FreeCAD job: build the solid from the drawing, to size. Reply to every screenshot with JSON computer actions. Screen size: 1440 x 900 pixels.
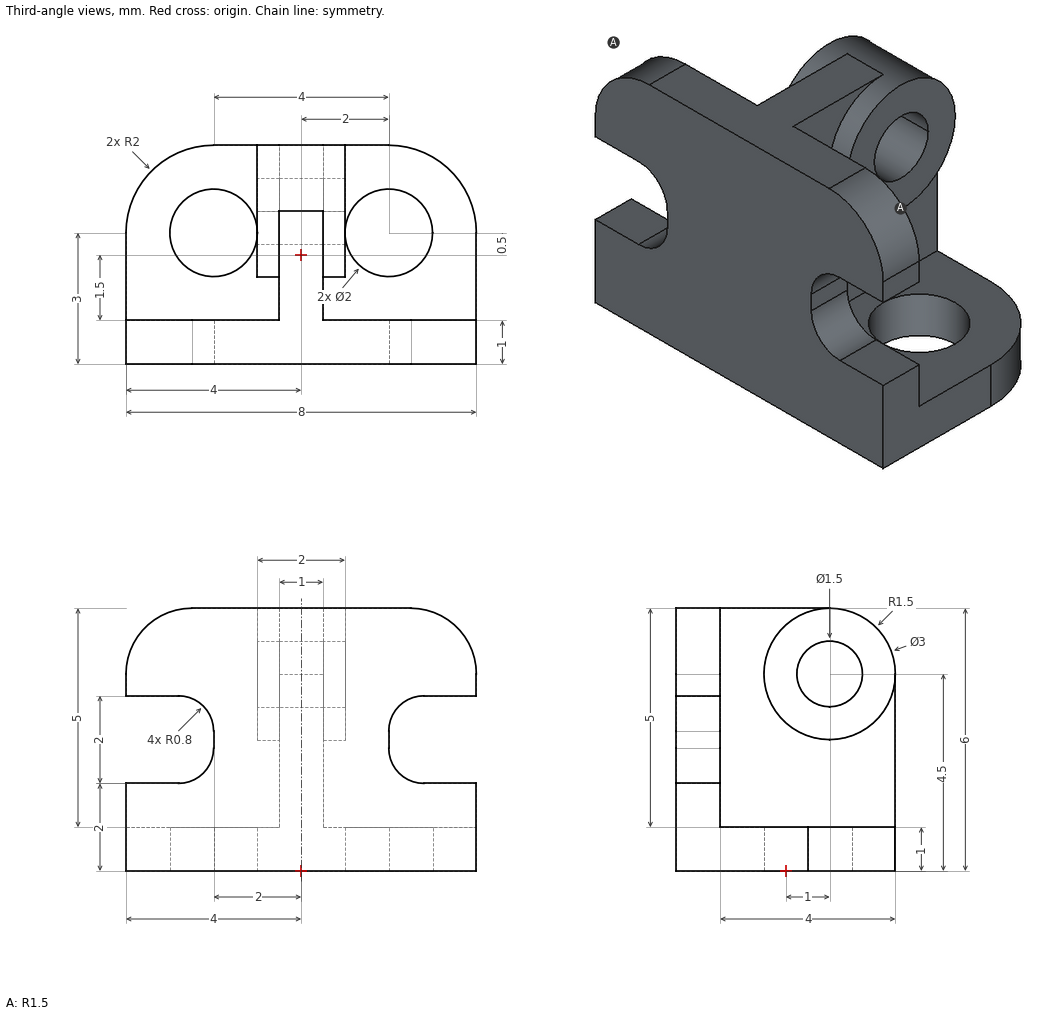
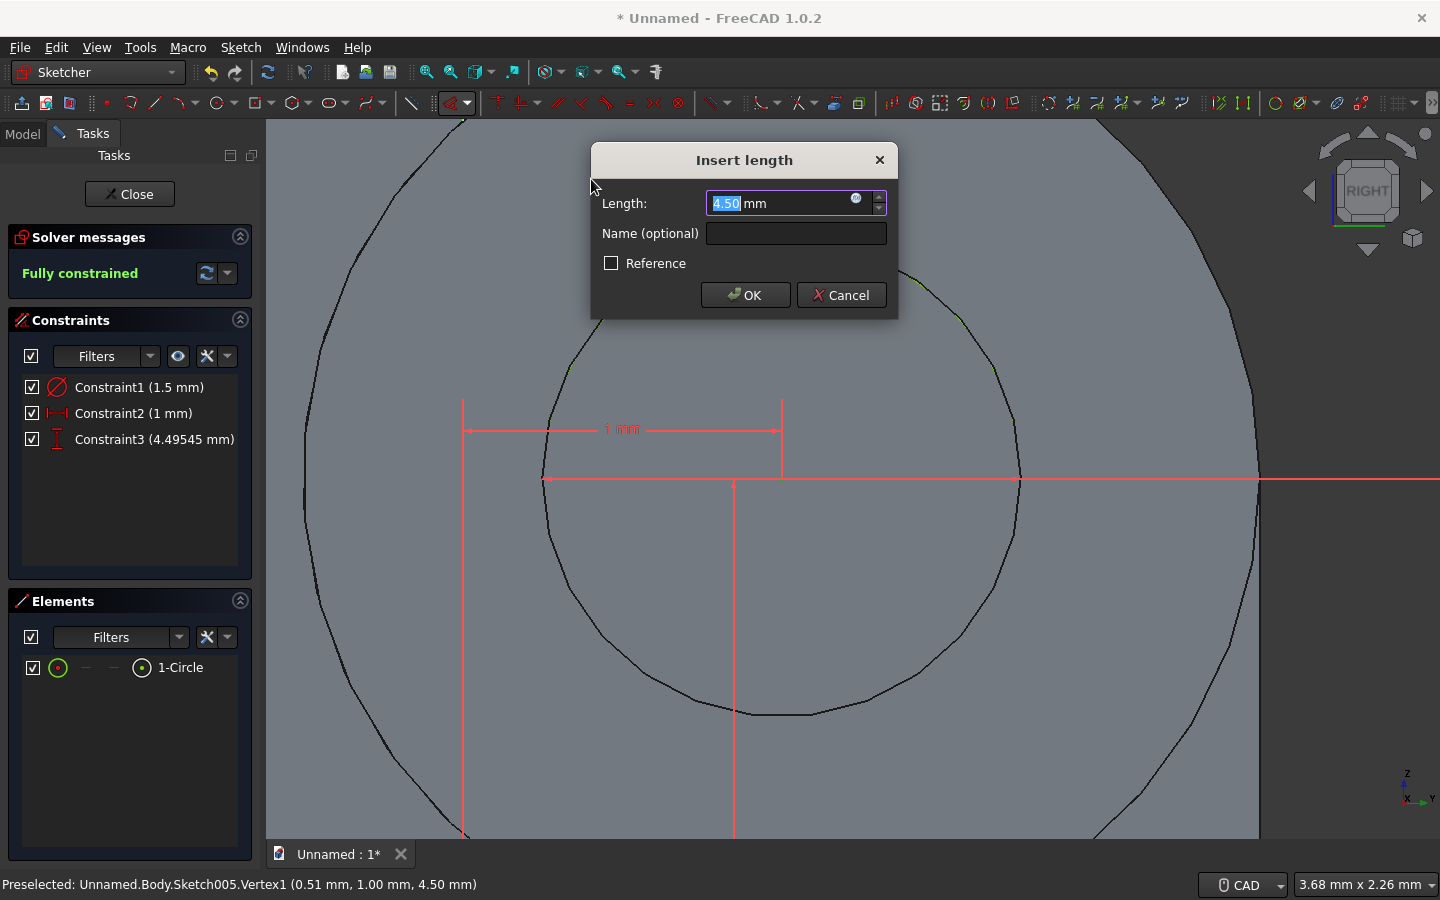
{"action": "type", "text": "4.5"}
{"action": "key", "text": "Return"}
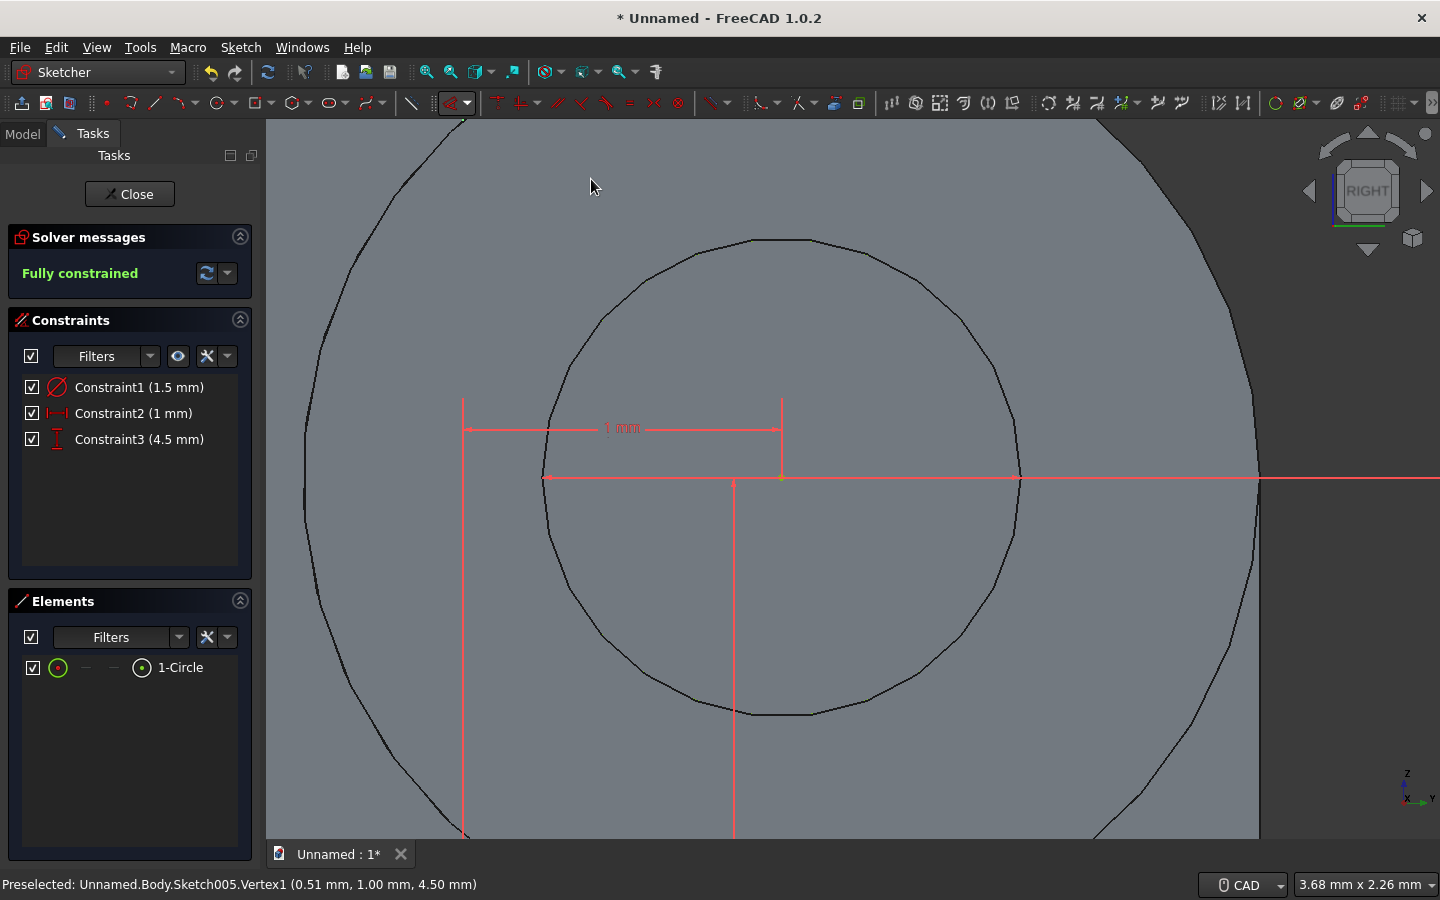
{"action": "left_click", "coordinate": [130, 194]}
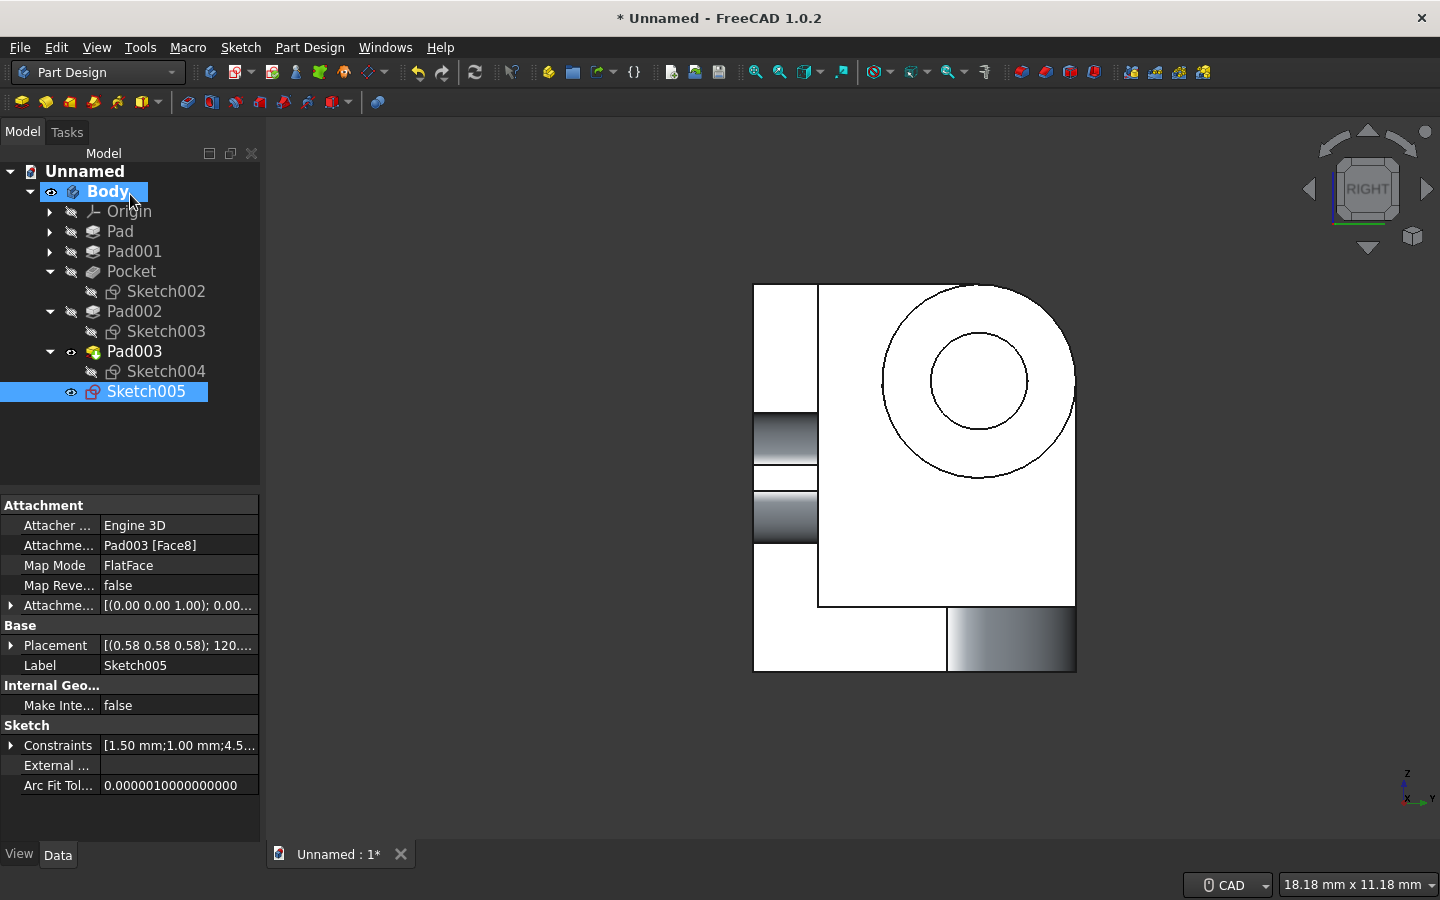
{"action": "left_click", "coordinate": [188, 102]}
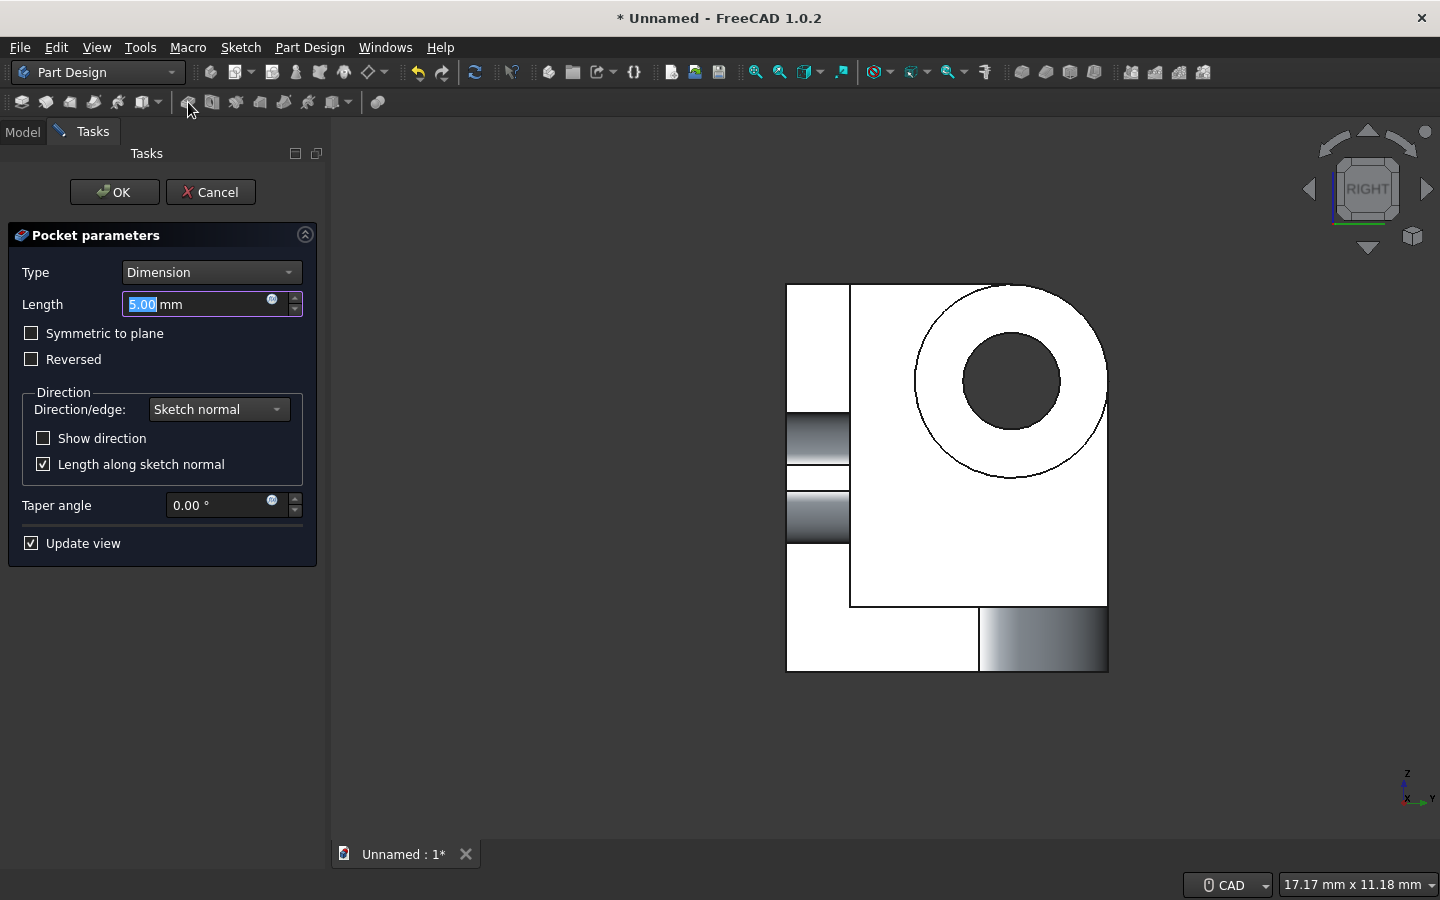
{"action": "left_click", "coordinate": [212, 272]}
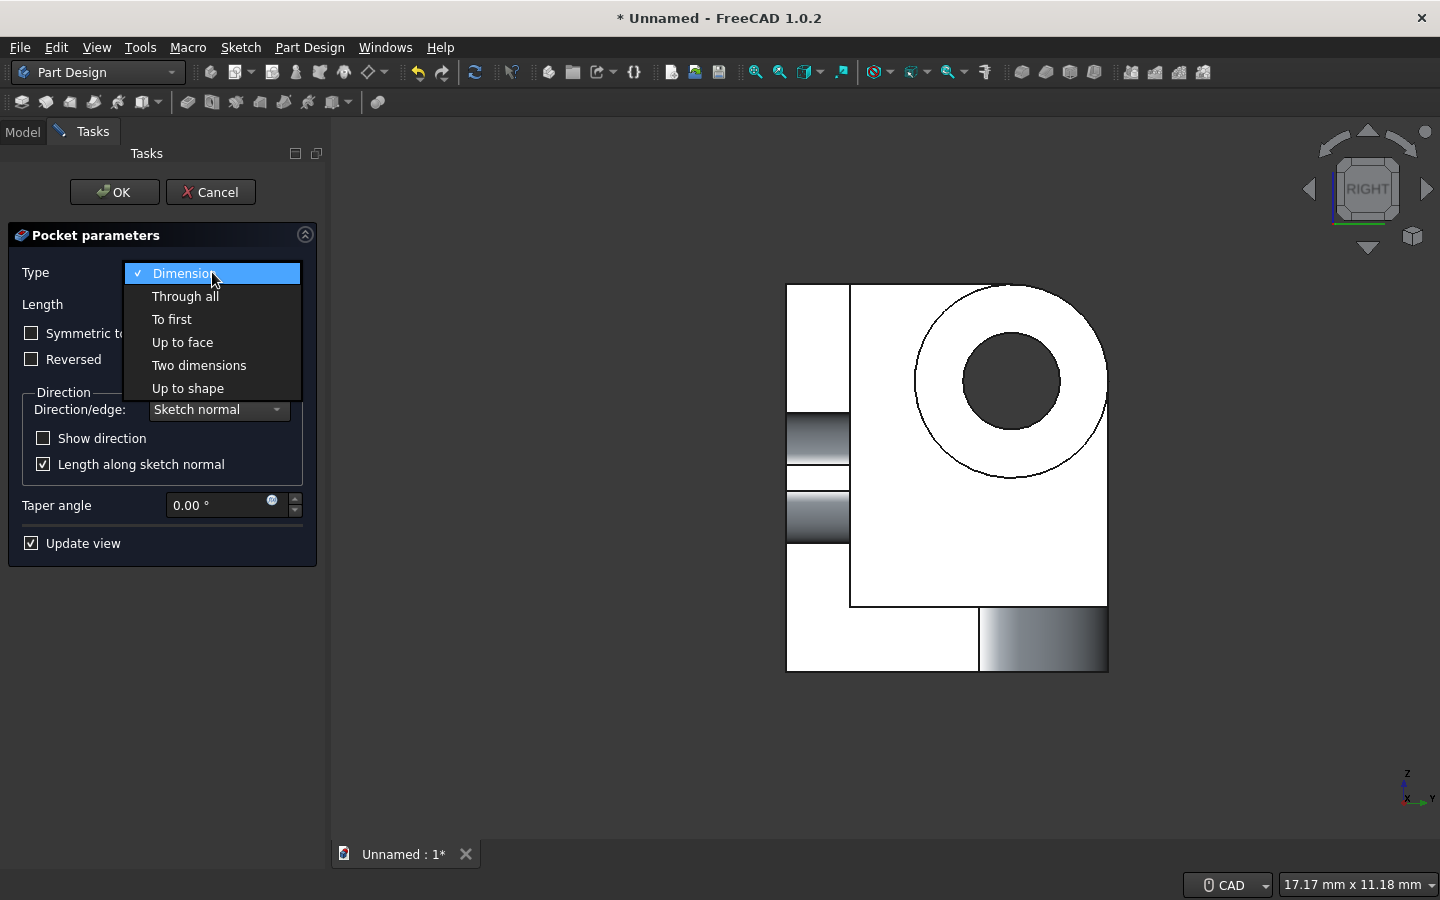
{"action": "left_click", "coordinate": [212, 296]}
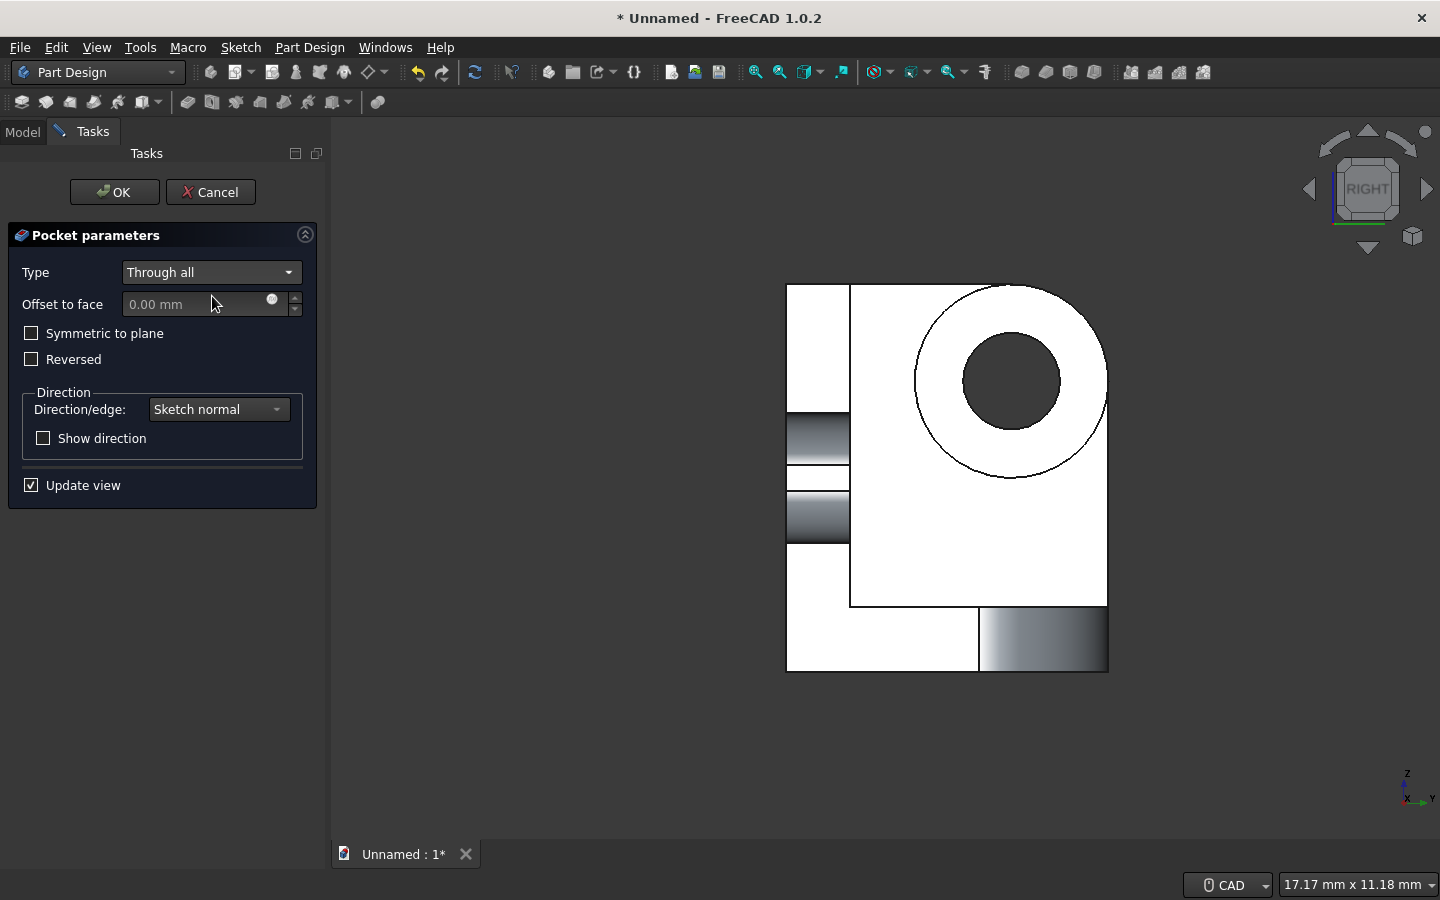
{"action": "left_click", "coordinate": [115, 192]}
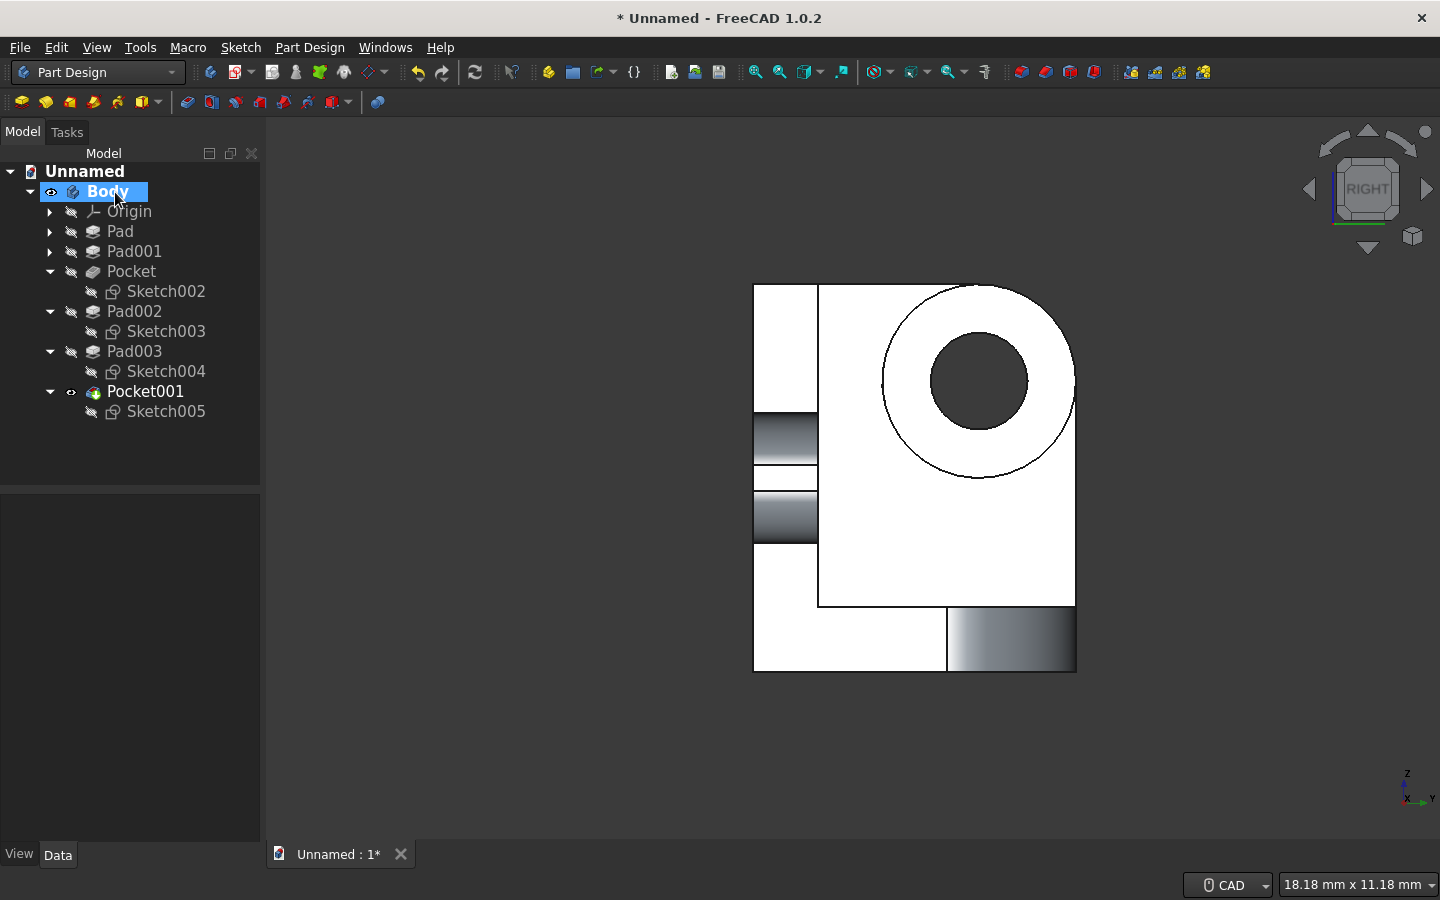
{"action": "key", "text": "0"}